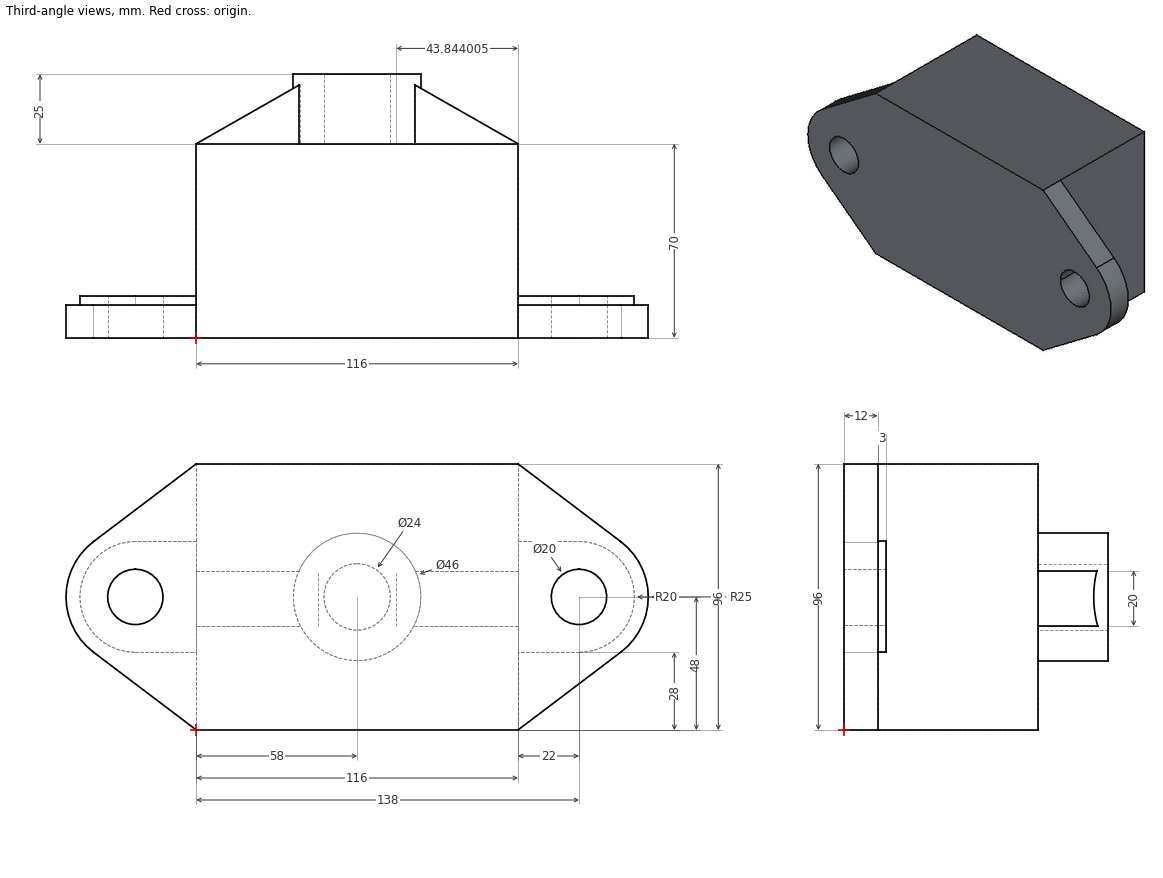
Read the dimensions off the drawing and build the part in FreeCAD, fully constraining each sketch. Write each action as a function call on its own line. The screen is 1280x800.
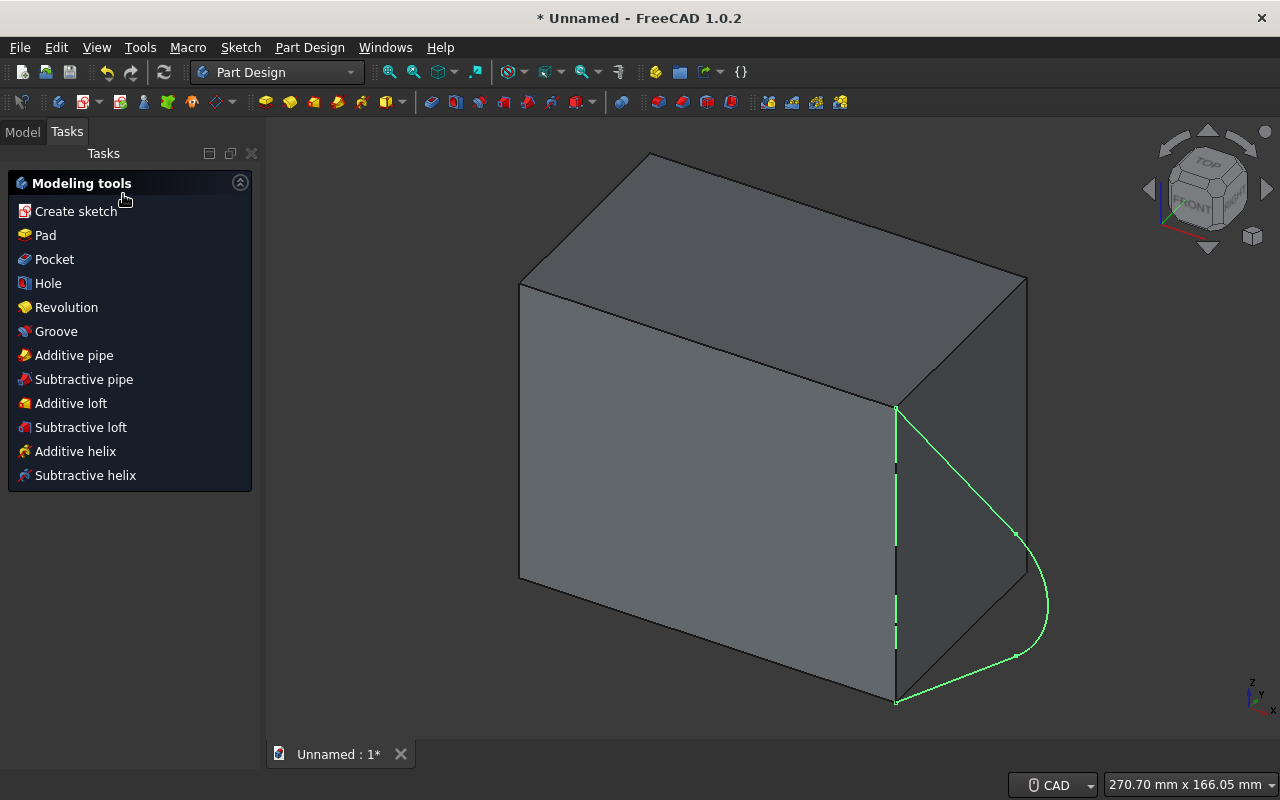
click(266, 102)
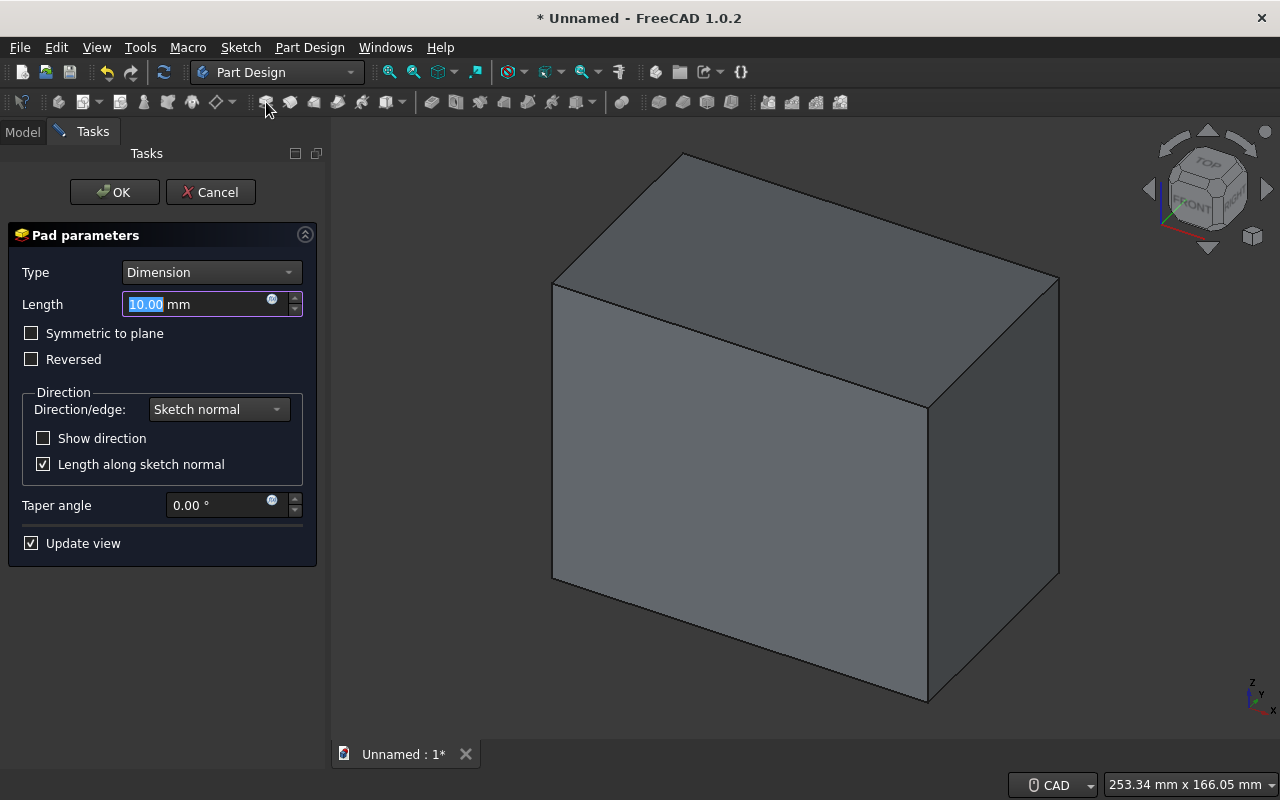
text(12)
key(Tab)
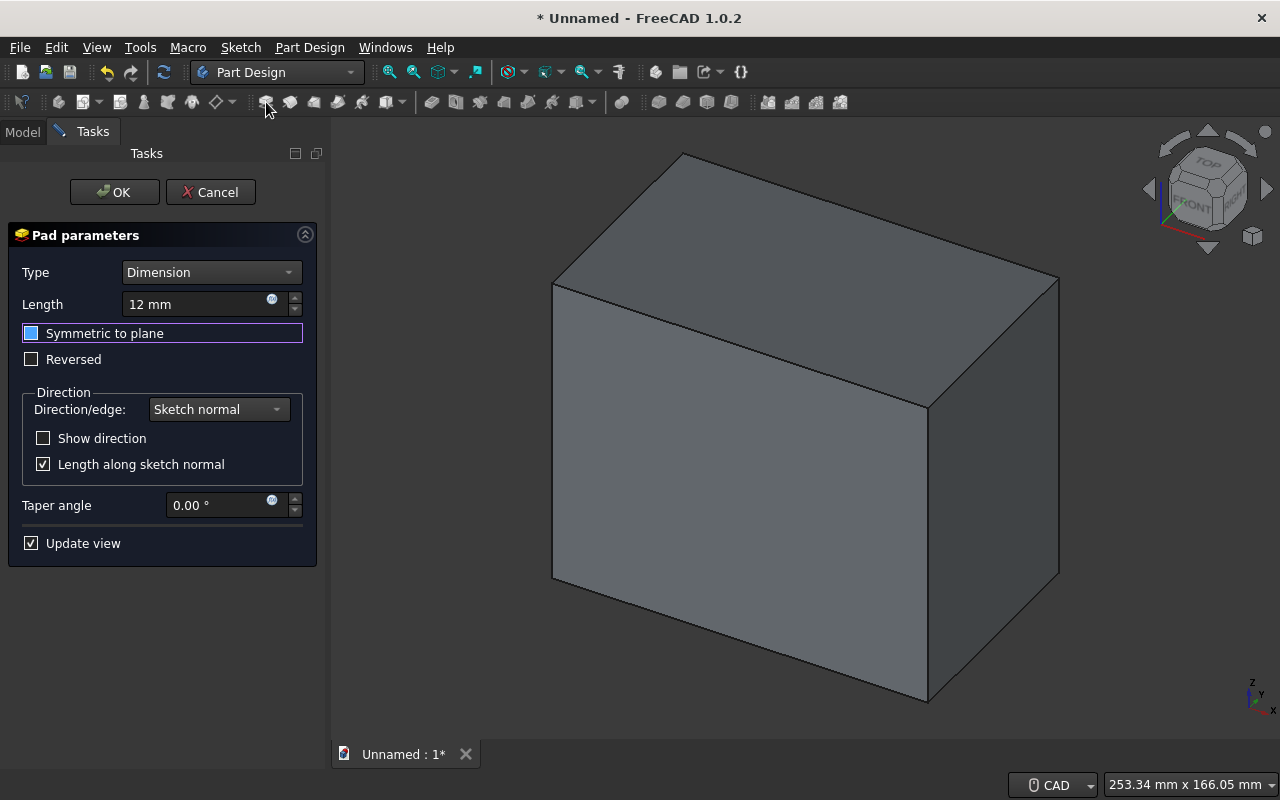
click(30, 359)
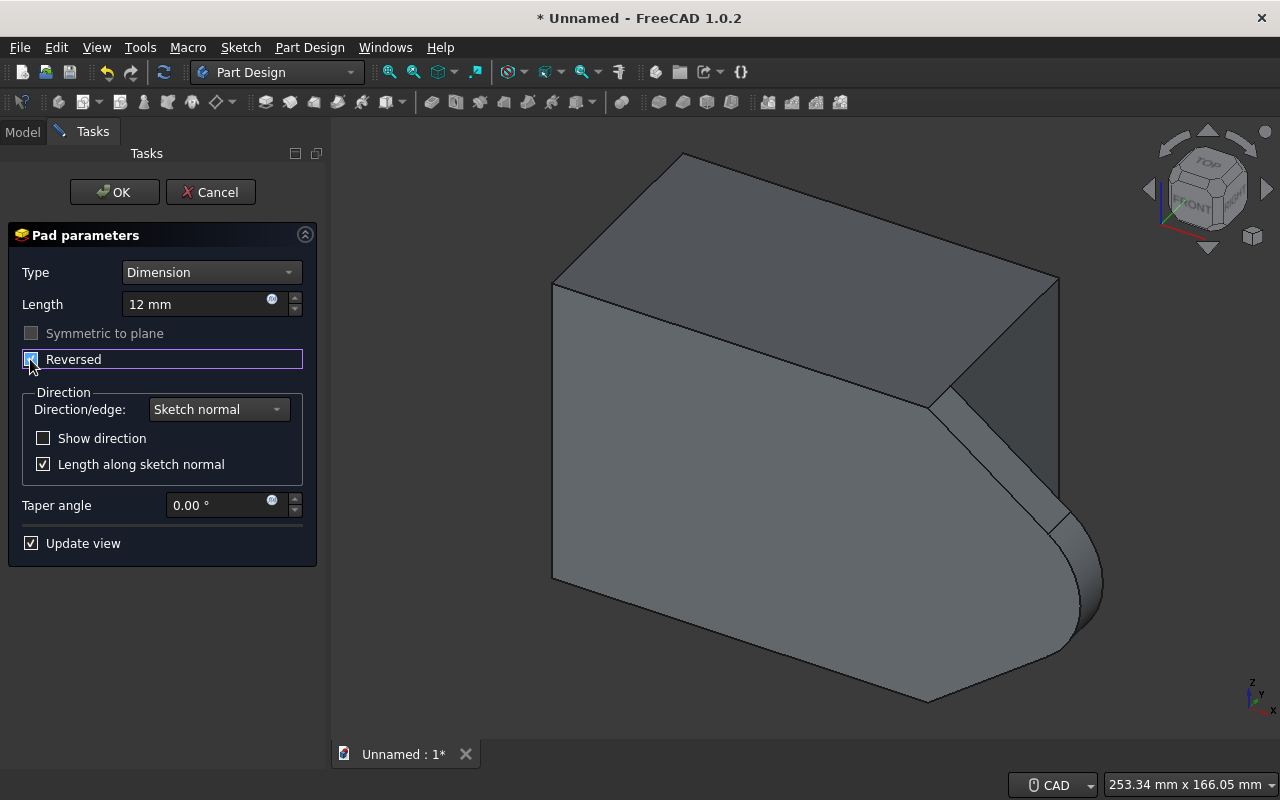
click(115, 192)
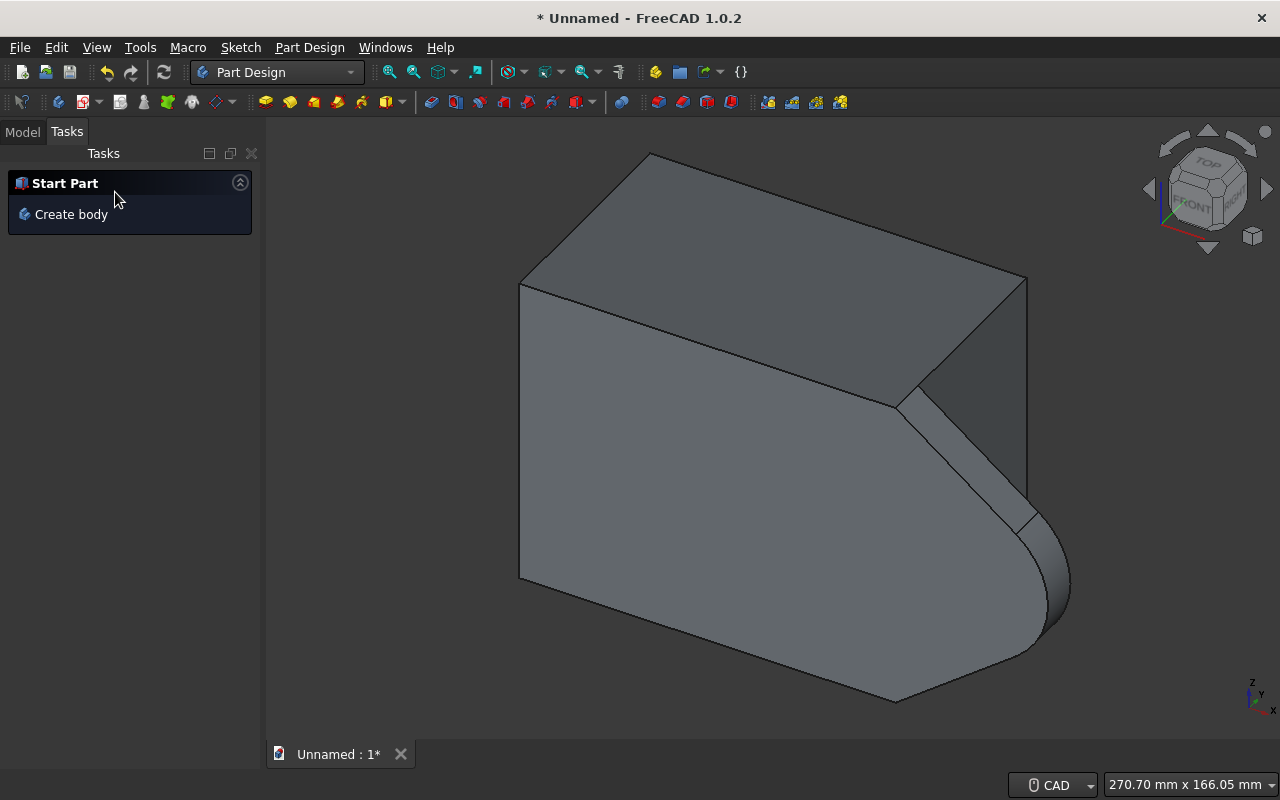
click(390, 72)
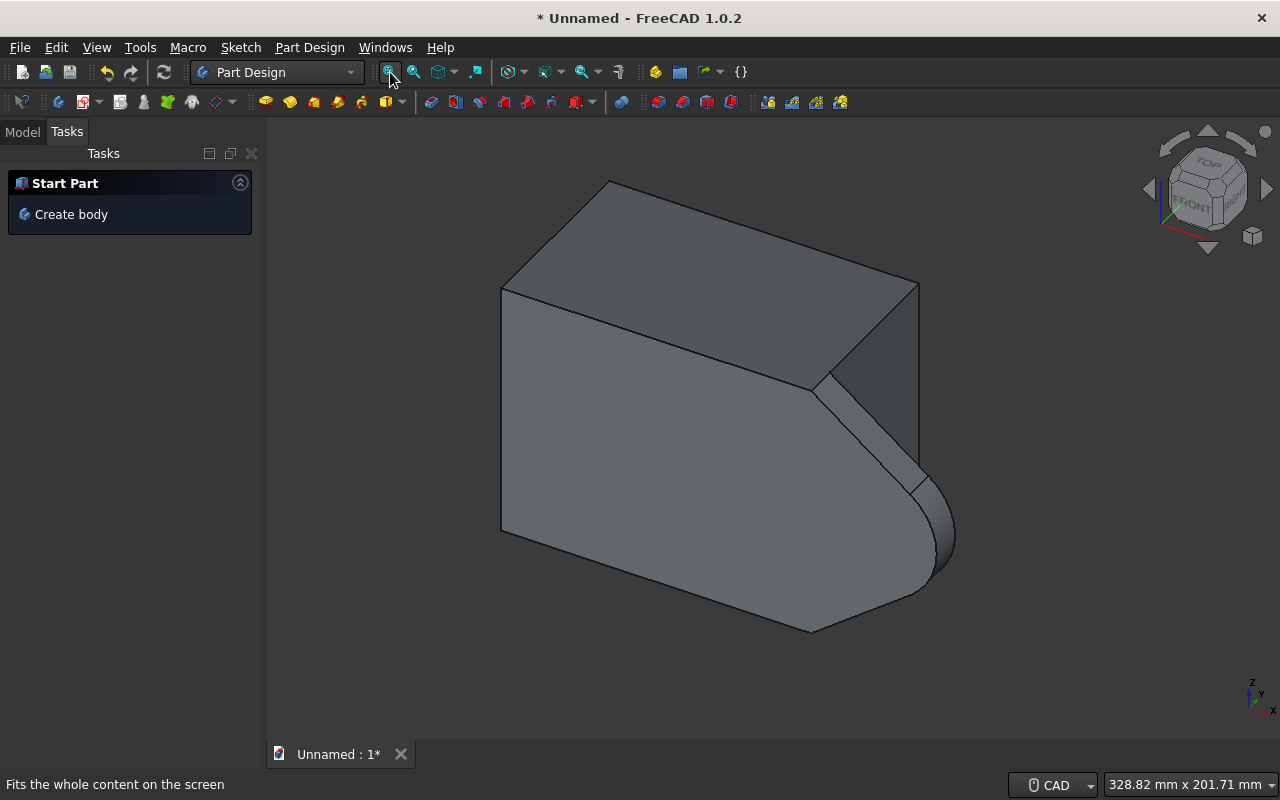
key(4)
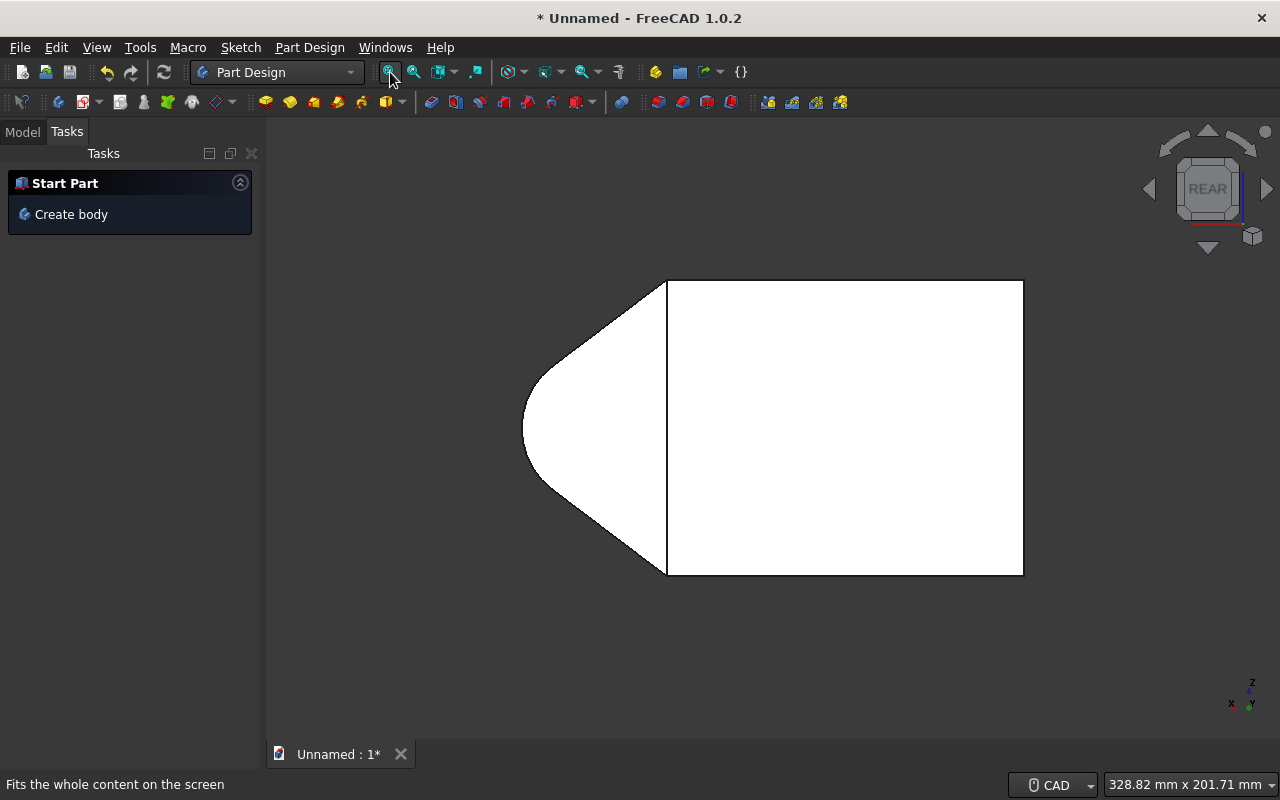
click(594, 427)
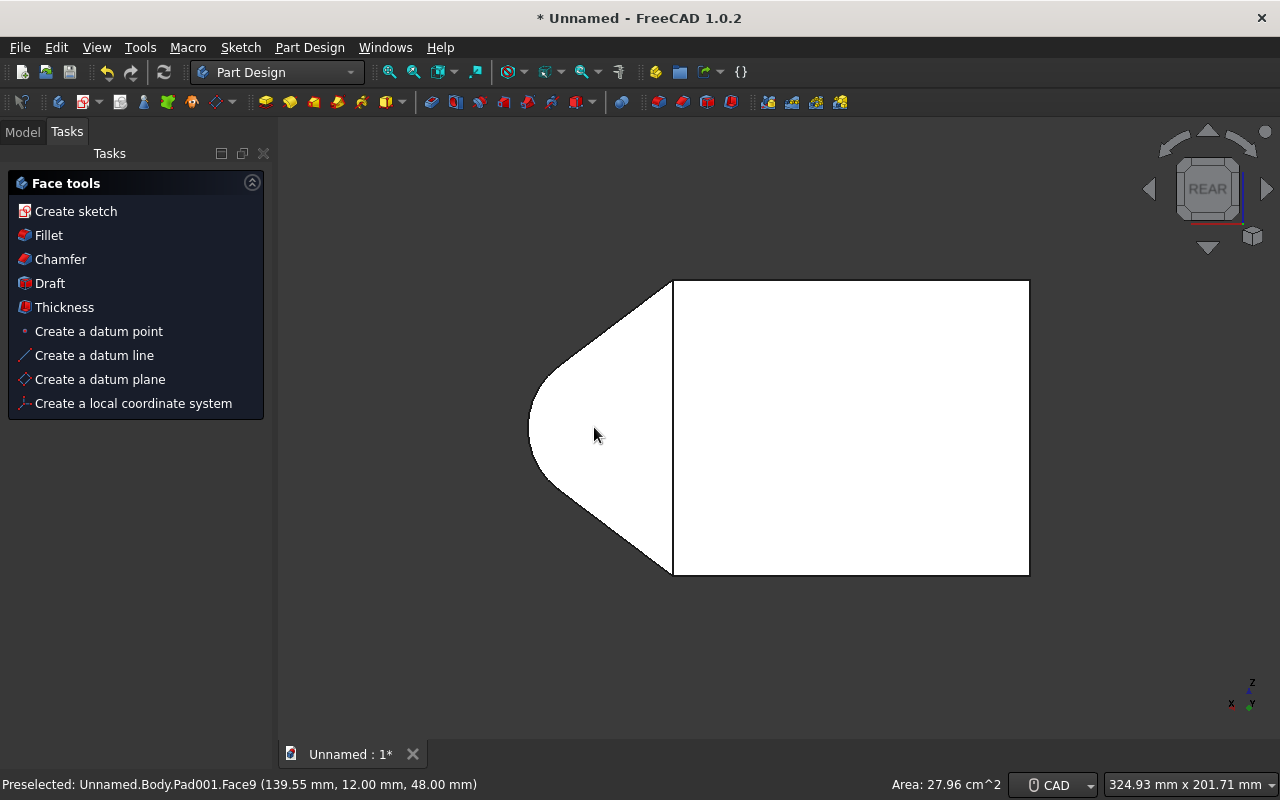
click(84, 102)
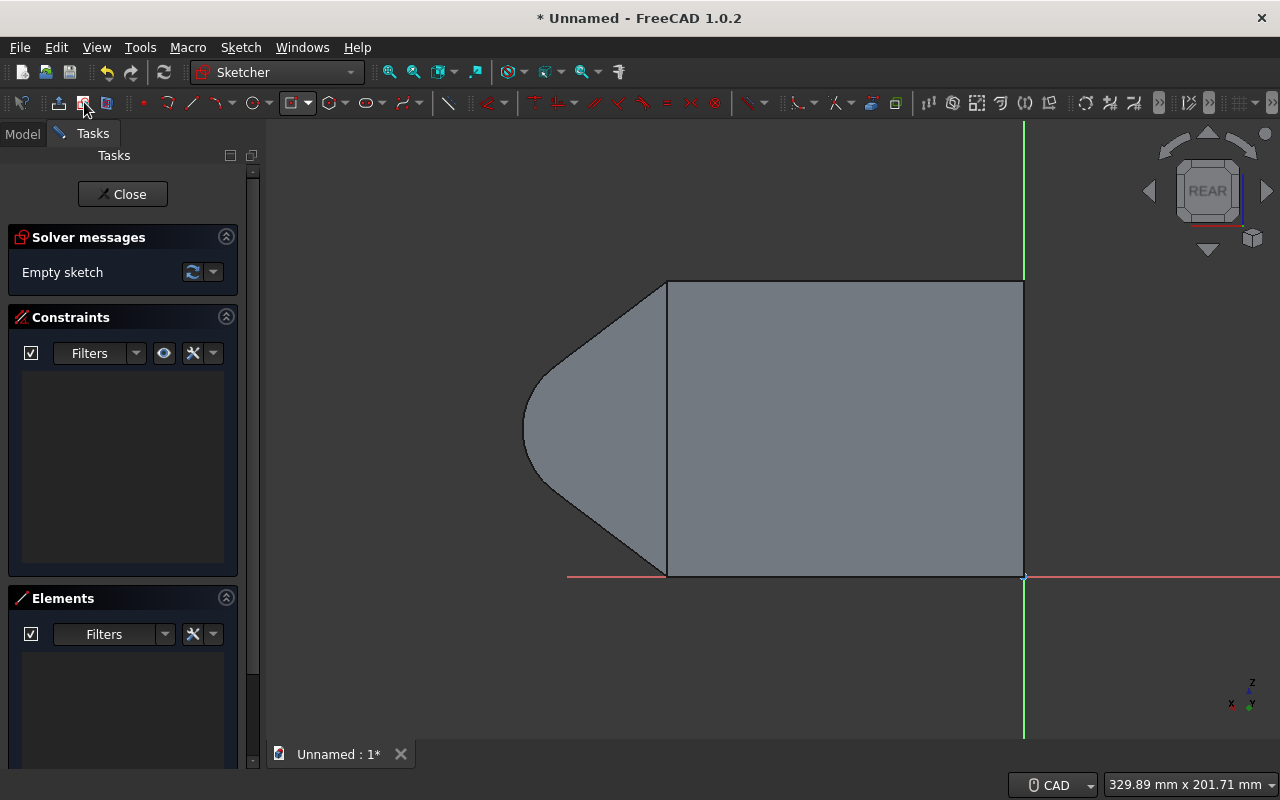
click(108, 104)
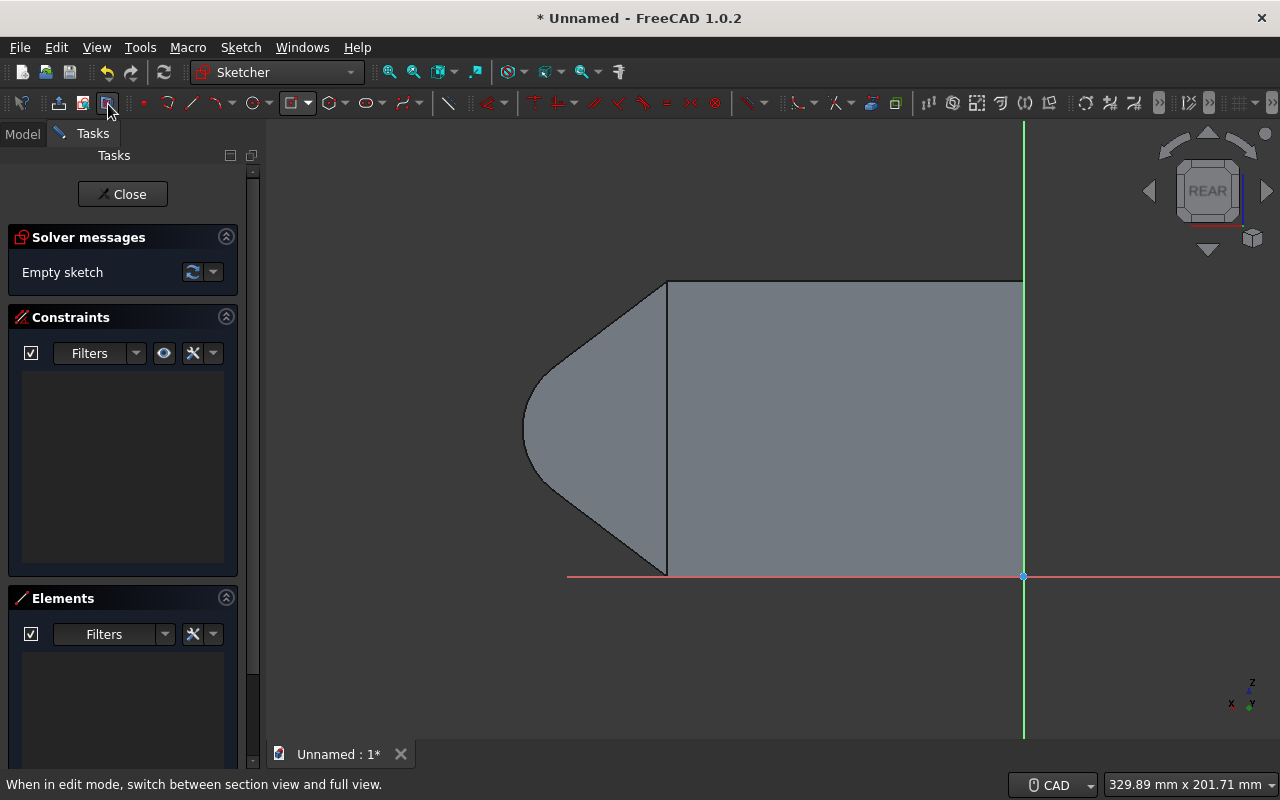
scroll(558, 429, up, 6)